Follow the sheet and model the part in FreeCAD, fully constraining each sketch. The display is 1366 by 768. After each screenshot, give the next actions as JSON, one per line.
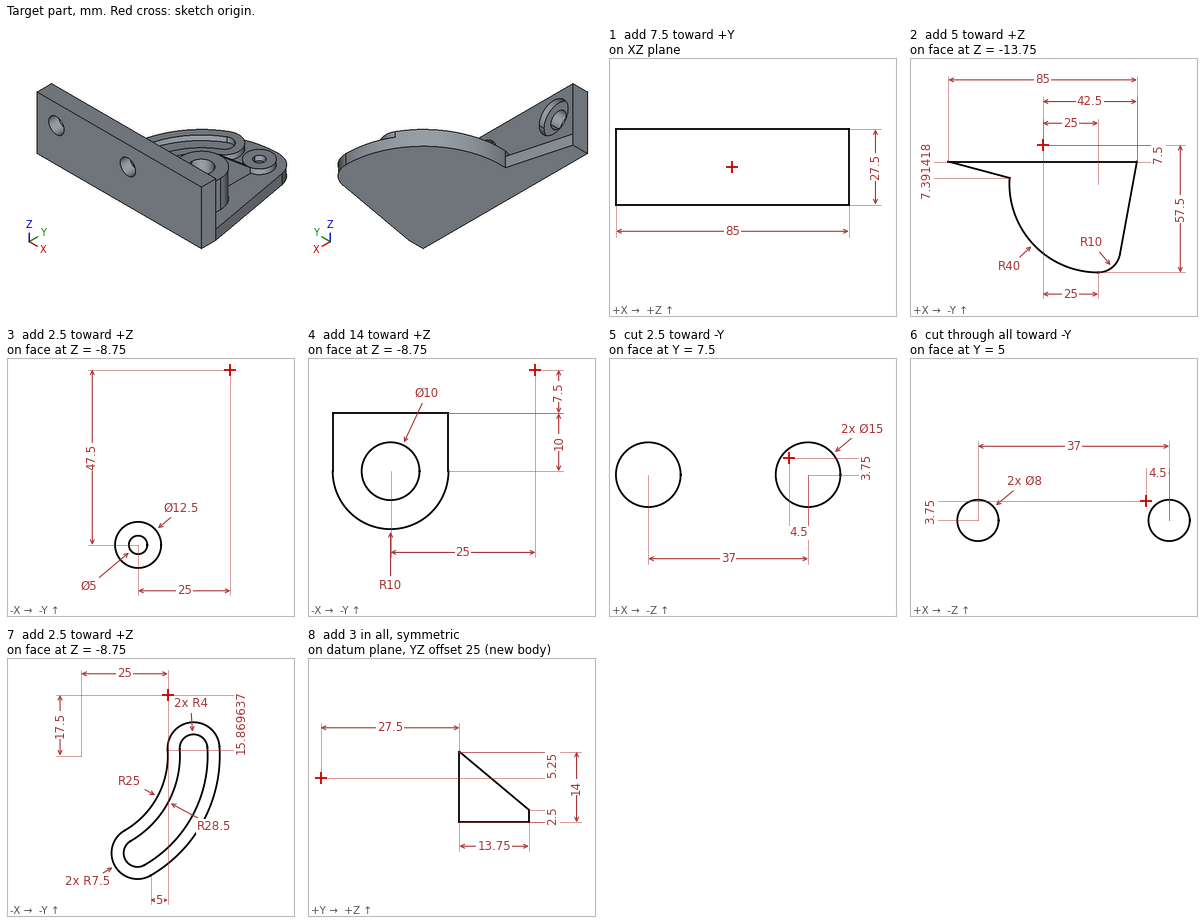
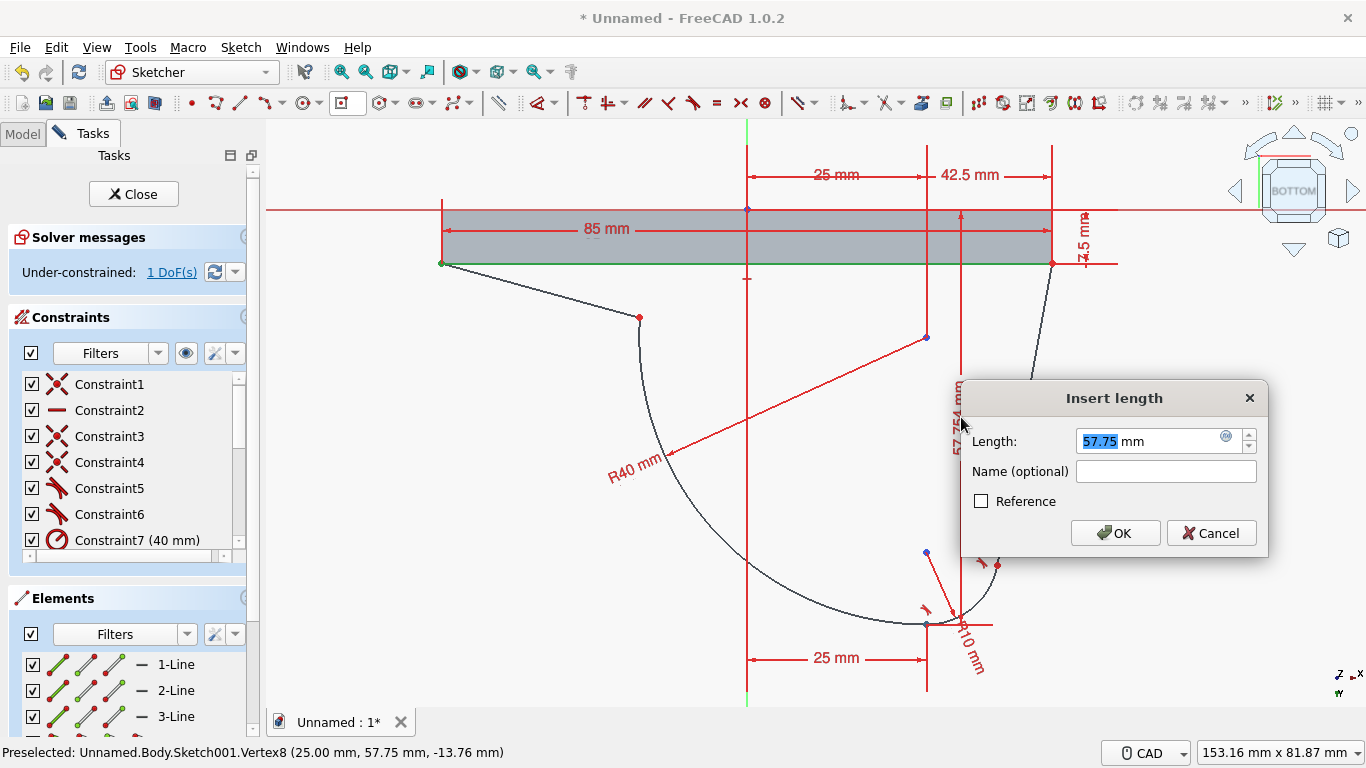
{"action": "type", "text": "57.5"}
{"action": "key", "text": "Return"}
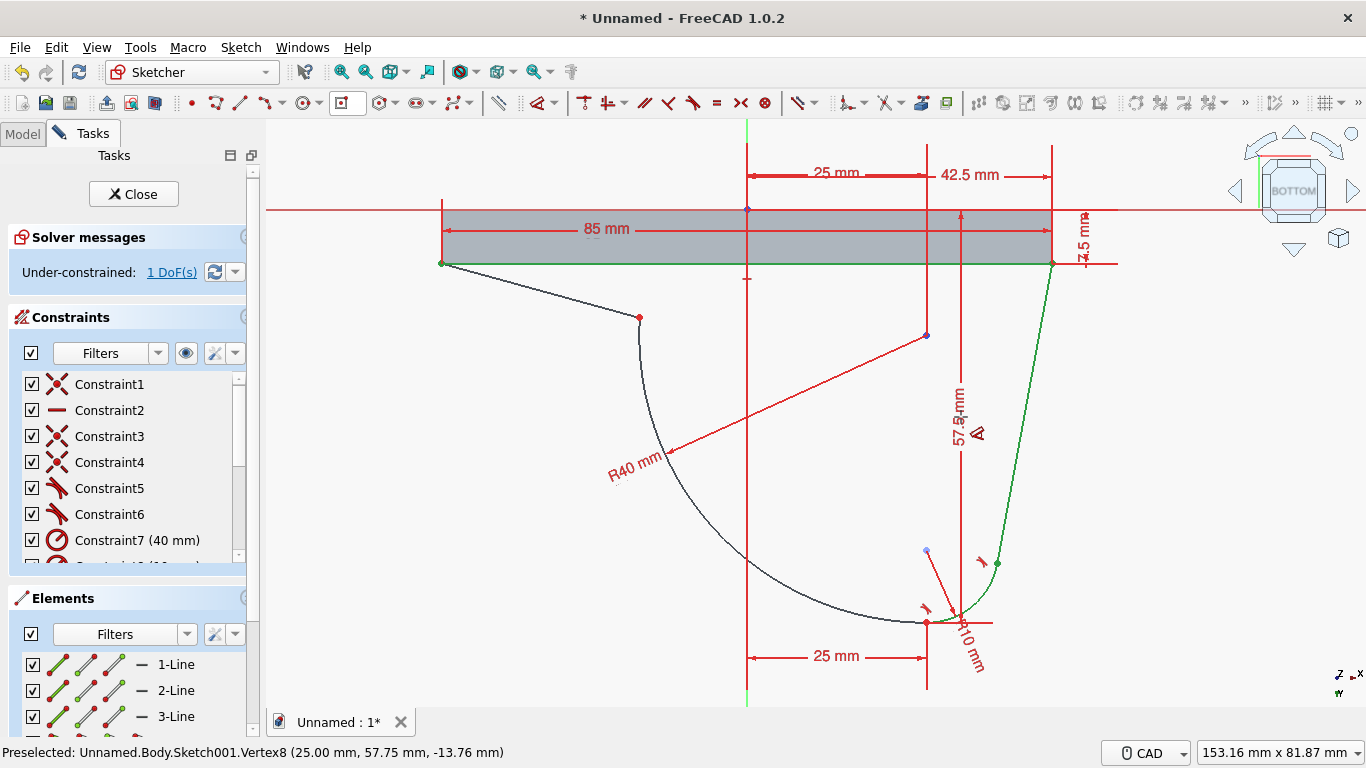
{"action": "left_click", "coordinate": [501, 280]}
{"action": "left_click", "coordinate": [408, 291]}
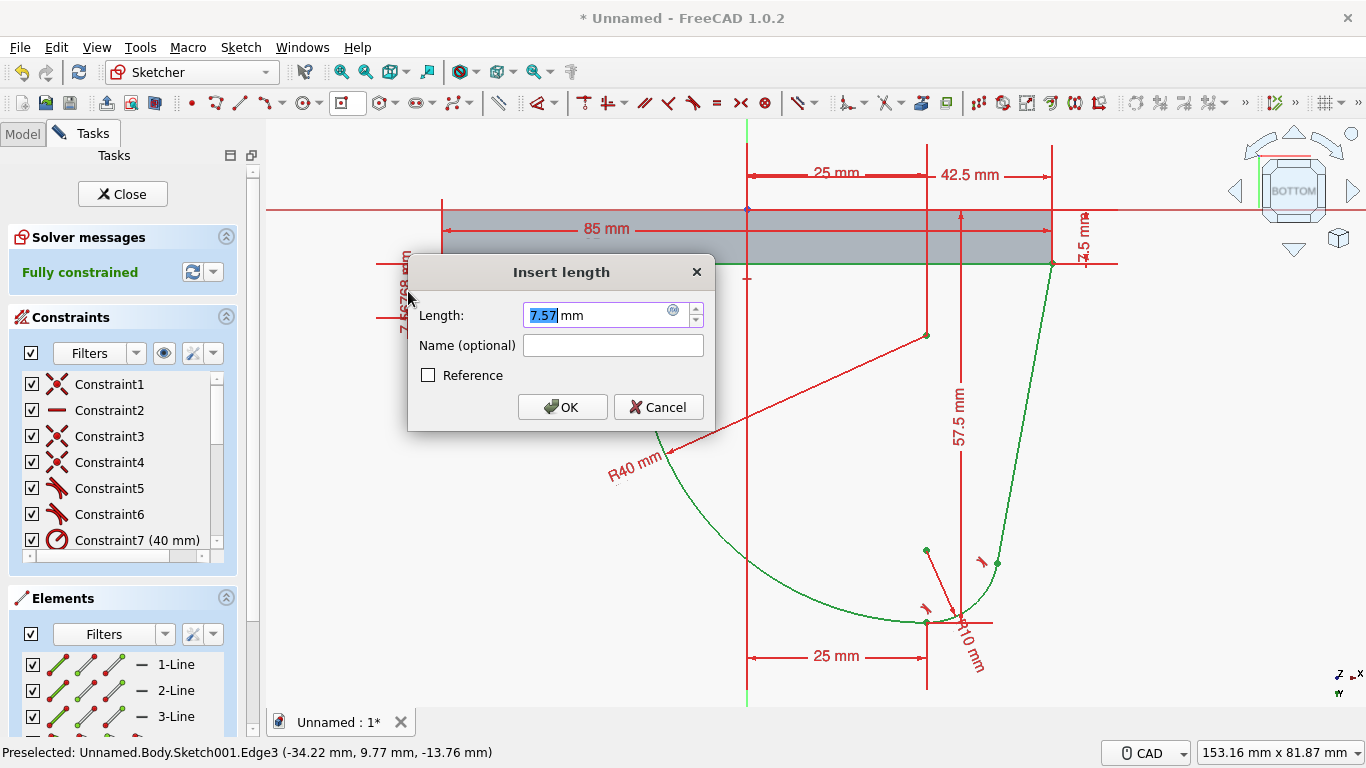
{"action": "type", "text": "7.391418"}
{"action": "key", "text": "Return"}
{"action": "key", "text": "Escape"}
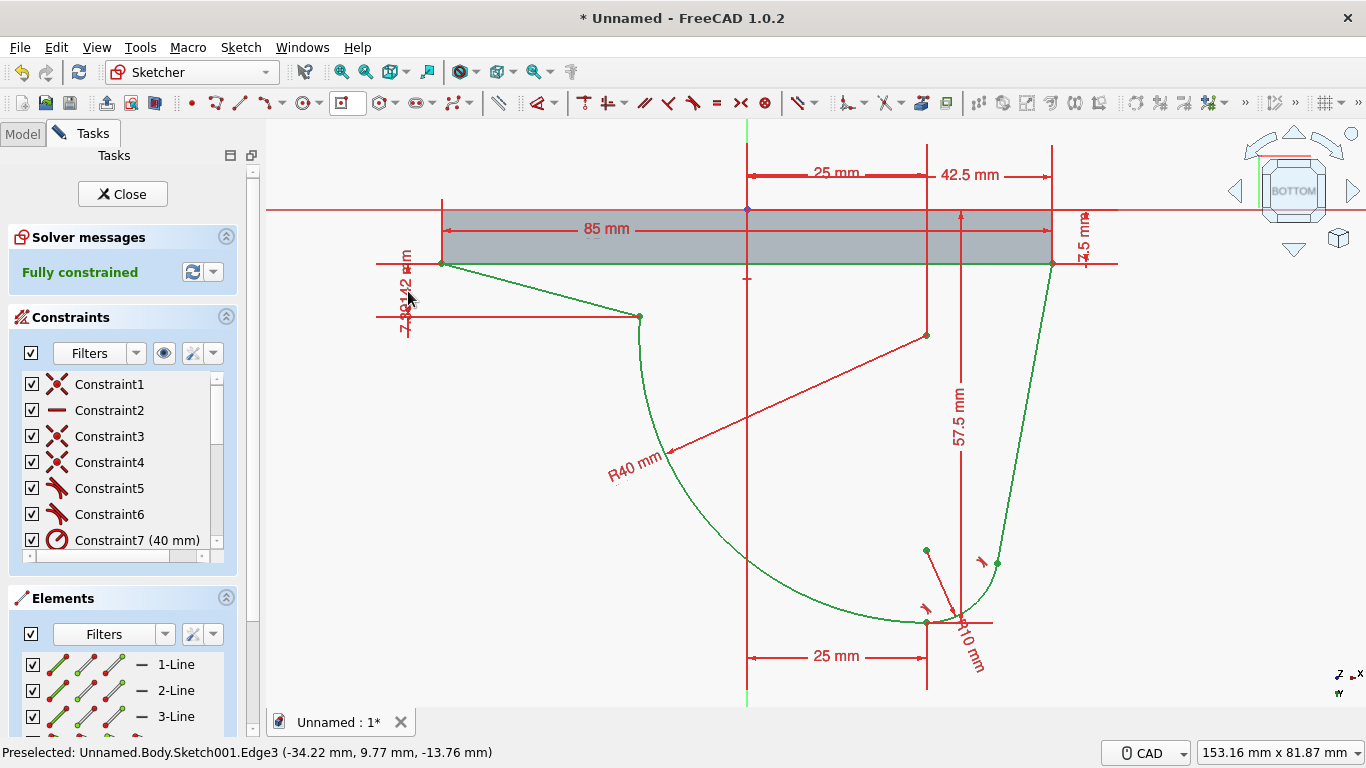
{"action": "left_click", "coordinate": [123, 194]}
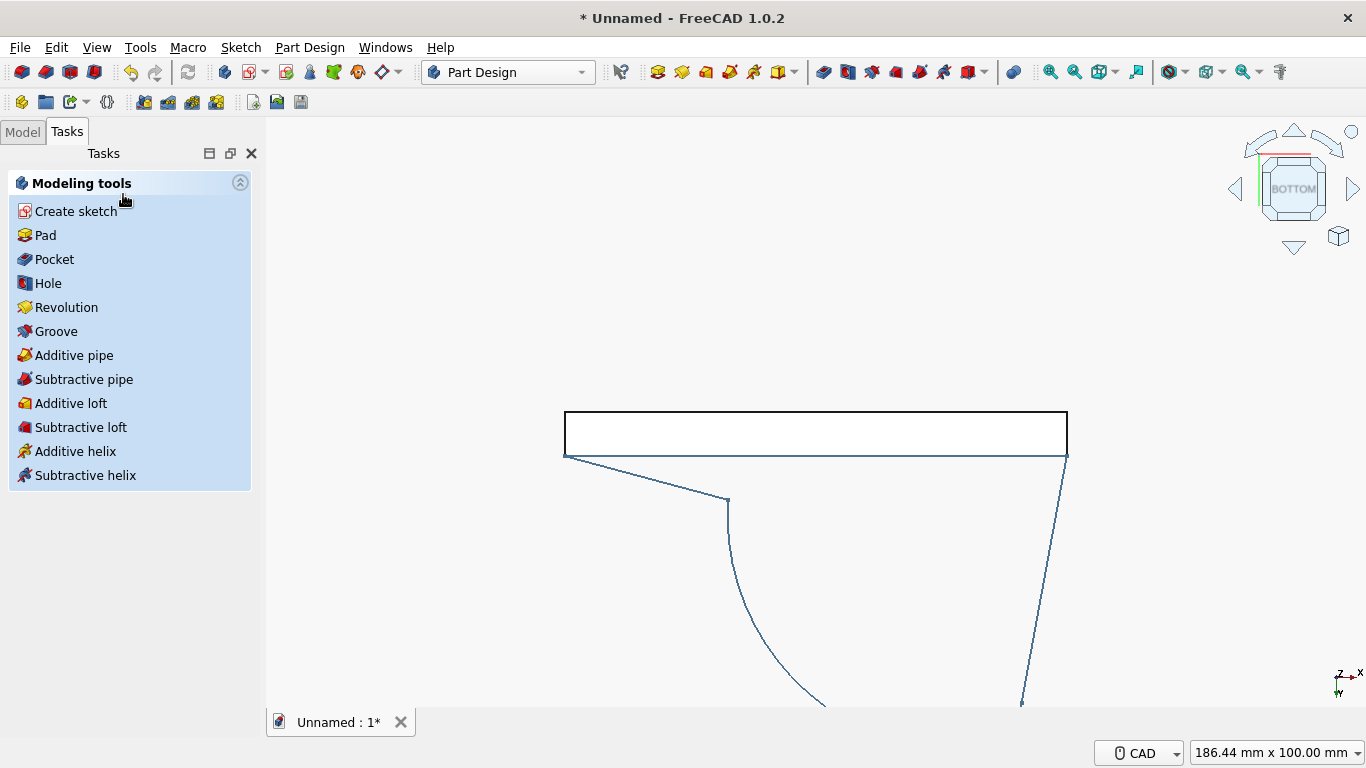
{"action": "left_click", "coordinate": [658, 72]}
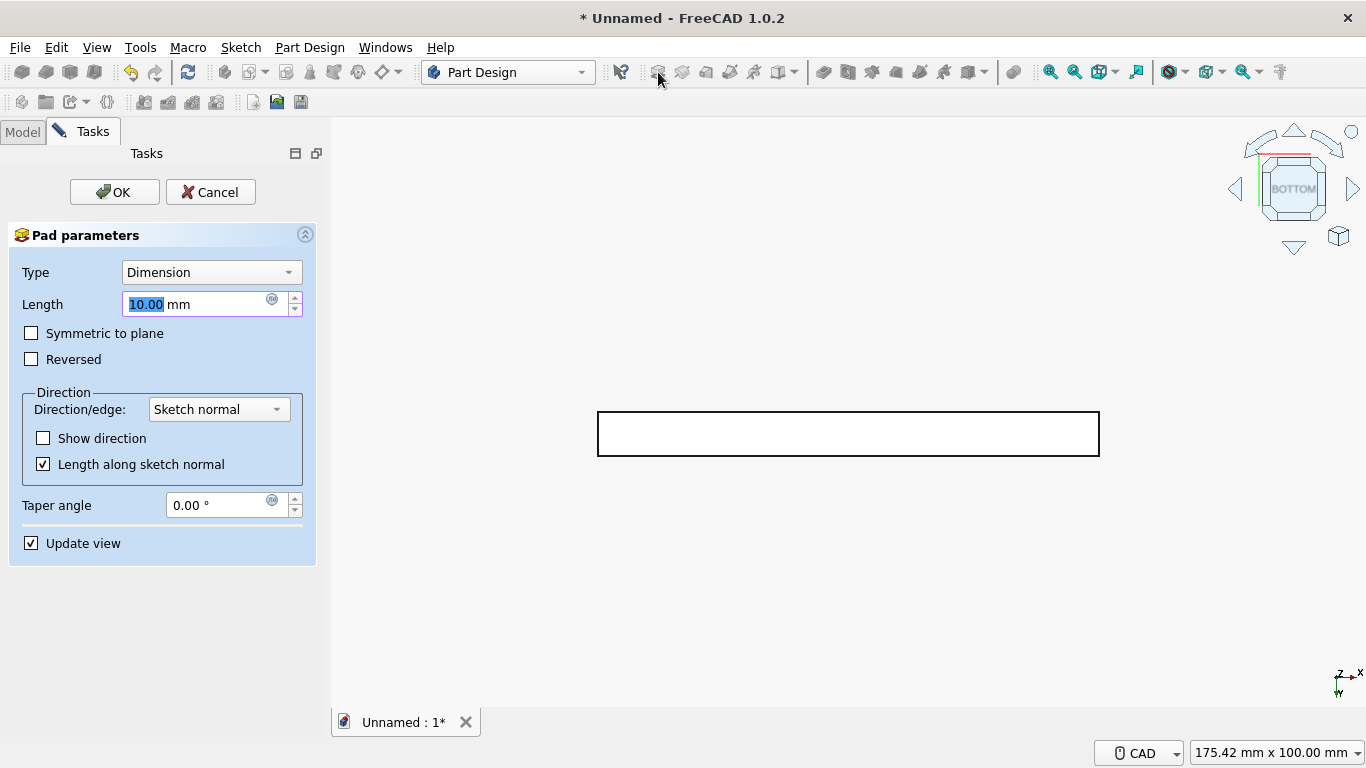
{"action": "type", "text": "5"}
{"action": "key", "text": "Tab"}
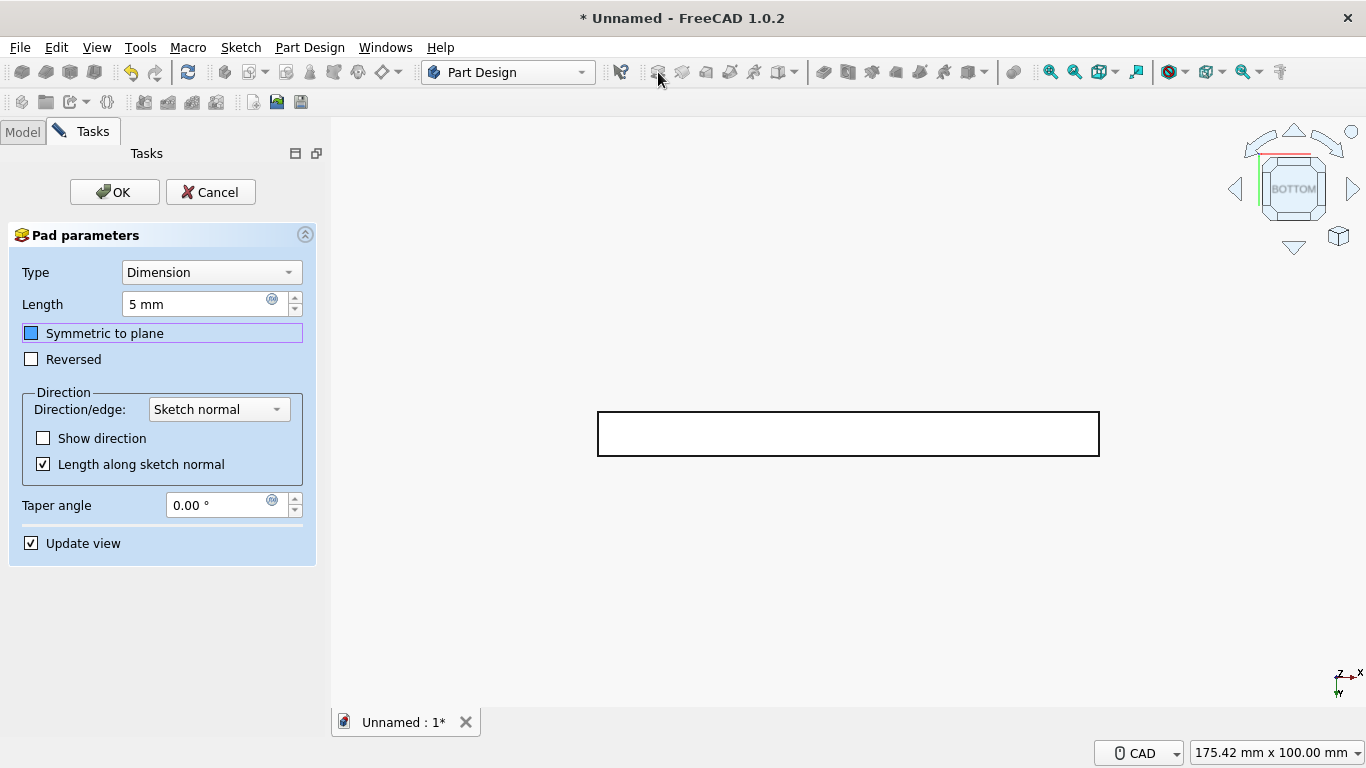
{"action": "left_click", "coordinate": [30, 359]}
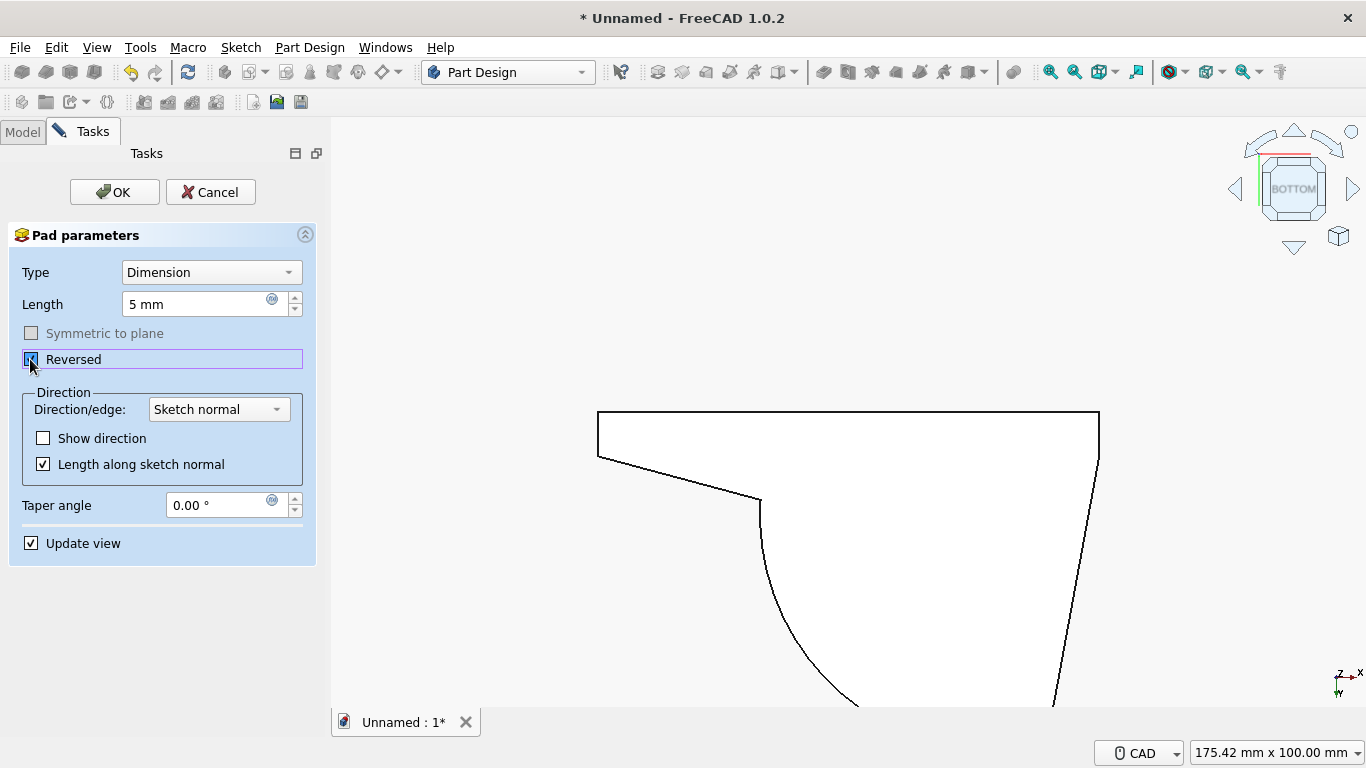
{"action": "left_click", "coordinate": [115, 192]}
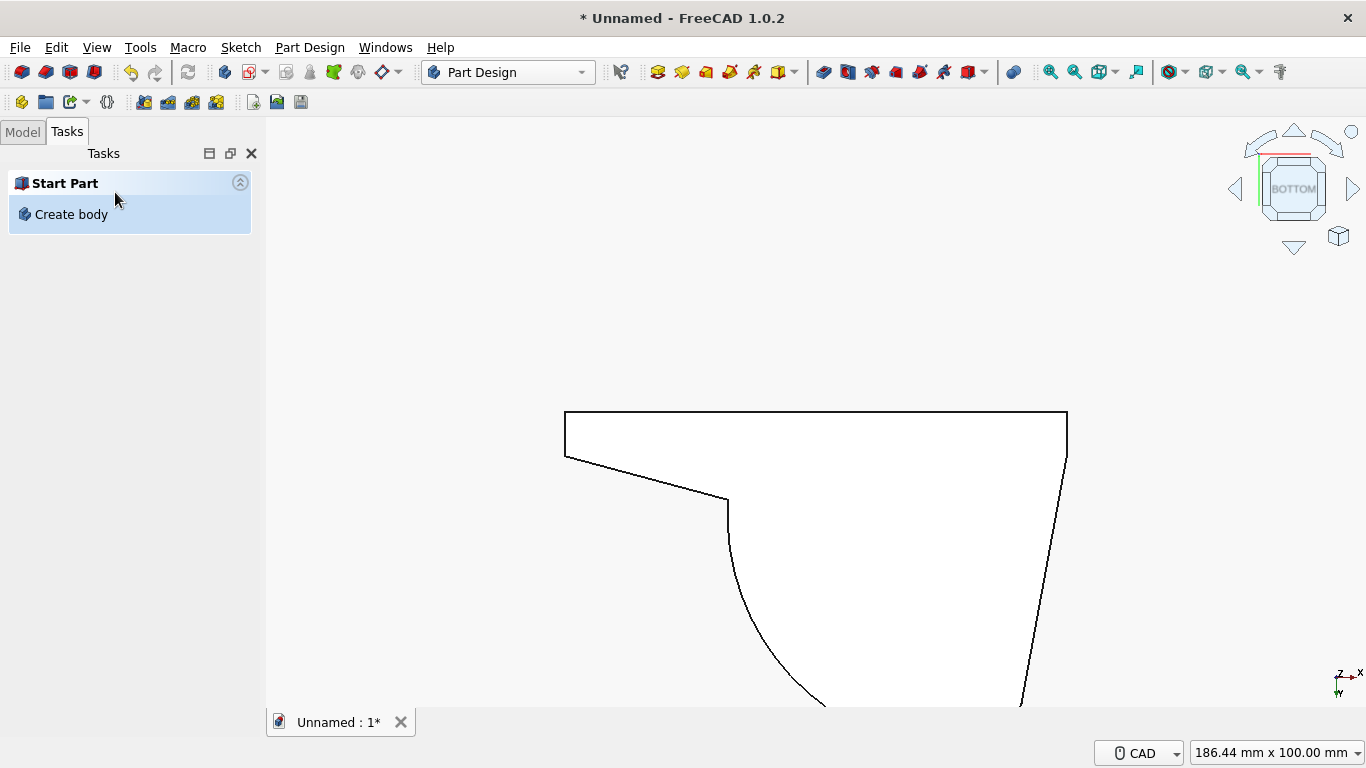
{"action": "left_click", "coordinate": [1052, 72]}